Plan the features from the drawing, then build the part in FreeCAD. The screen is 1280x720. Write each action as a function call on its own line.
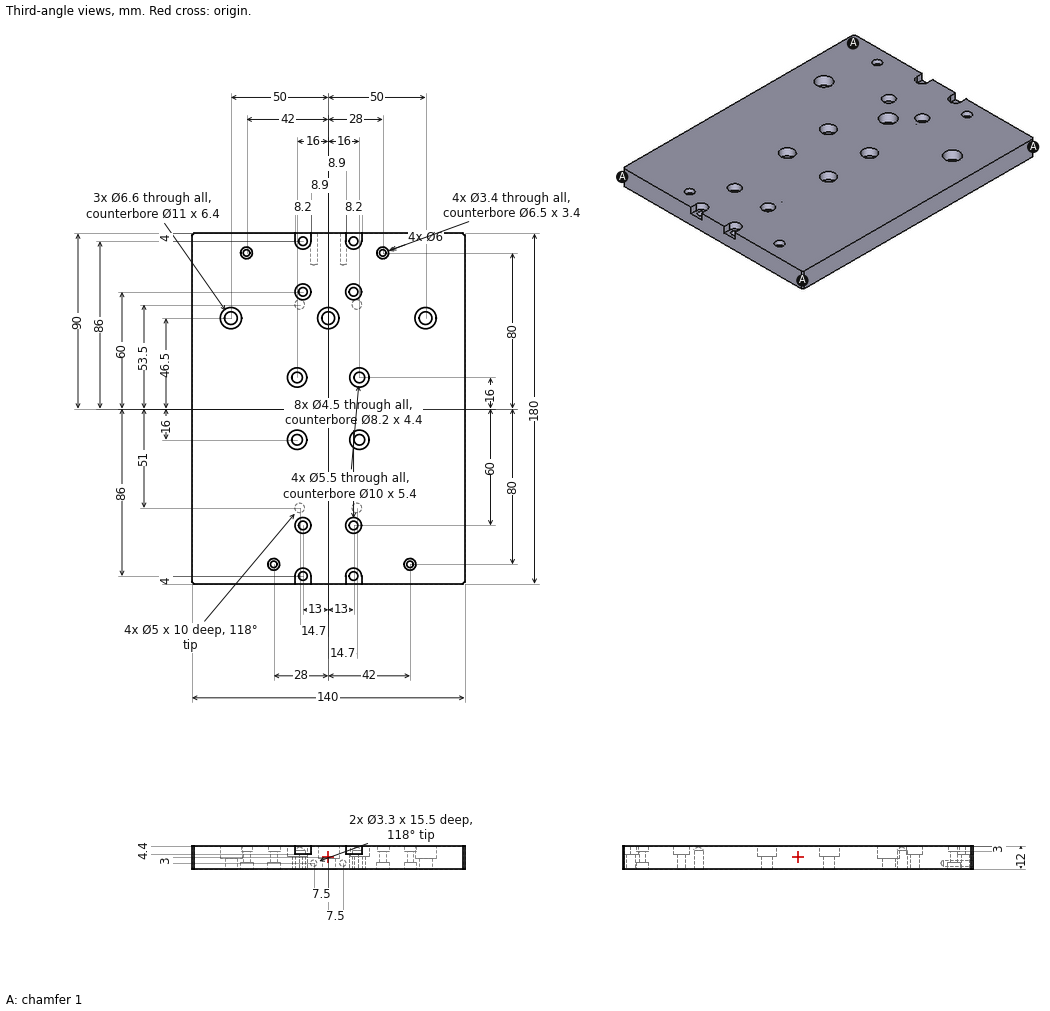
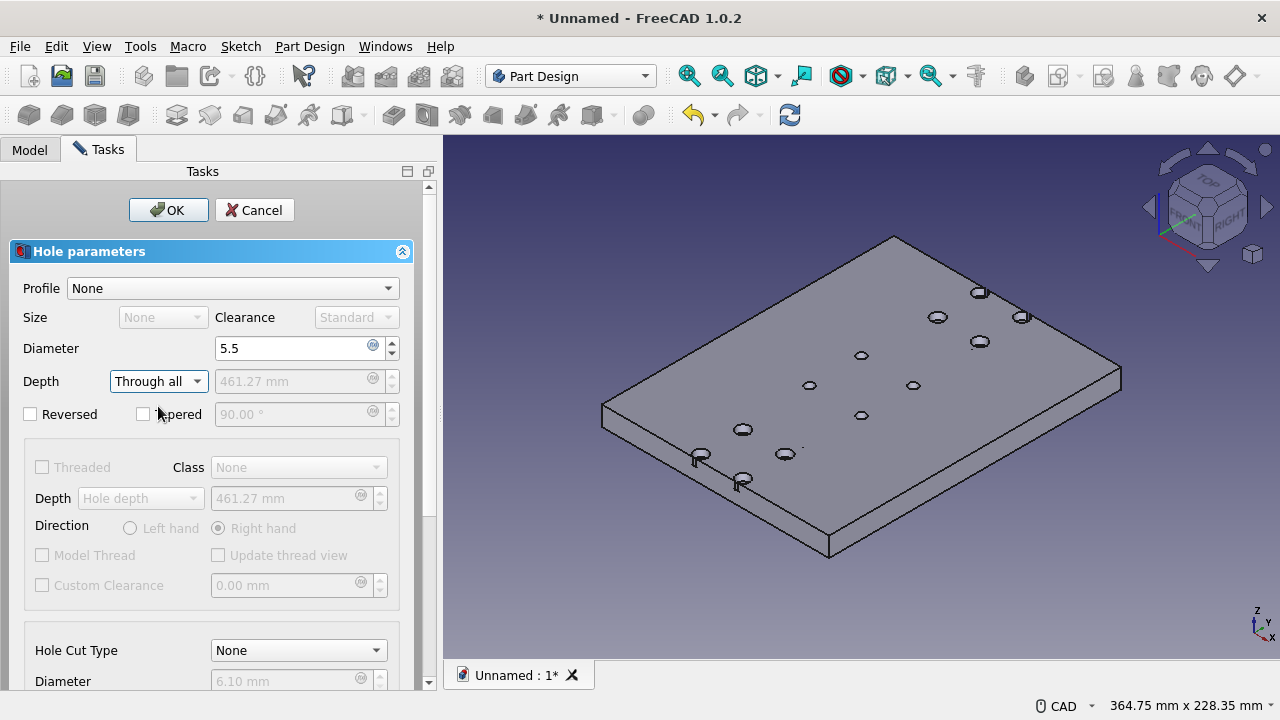
click(300, 650)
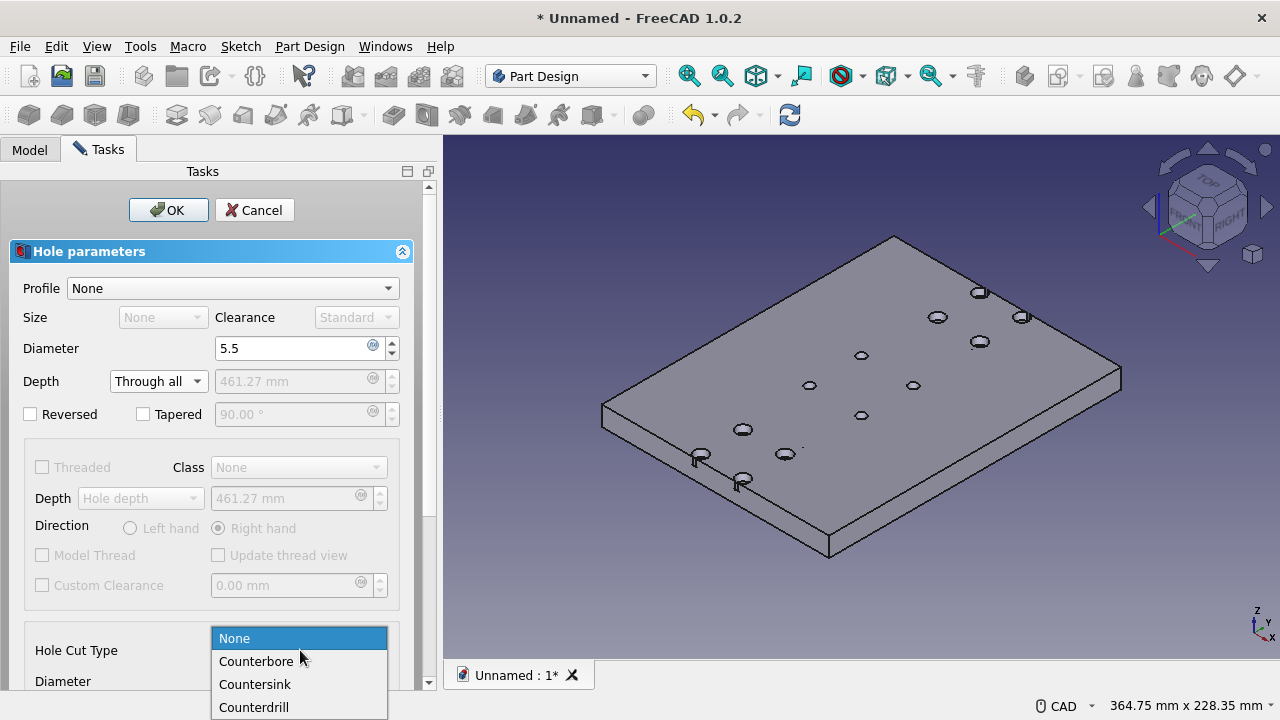
click(298, 662)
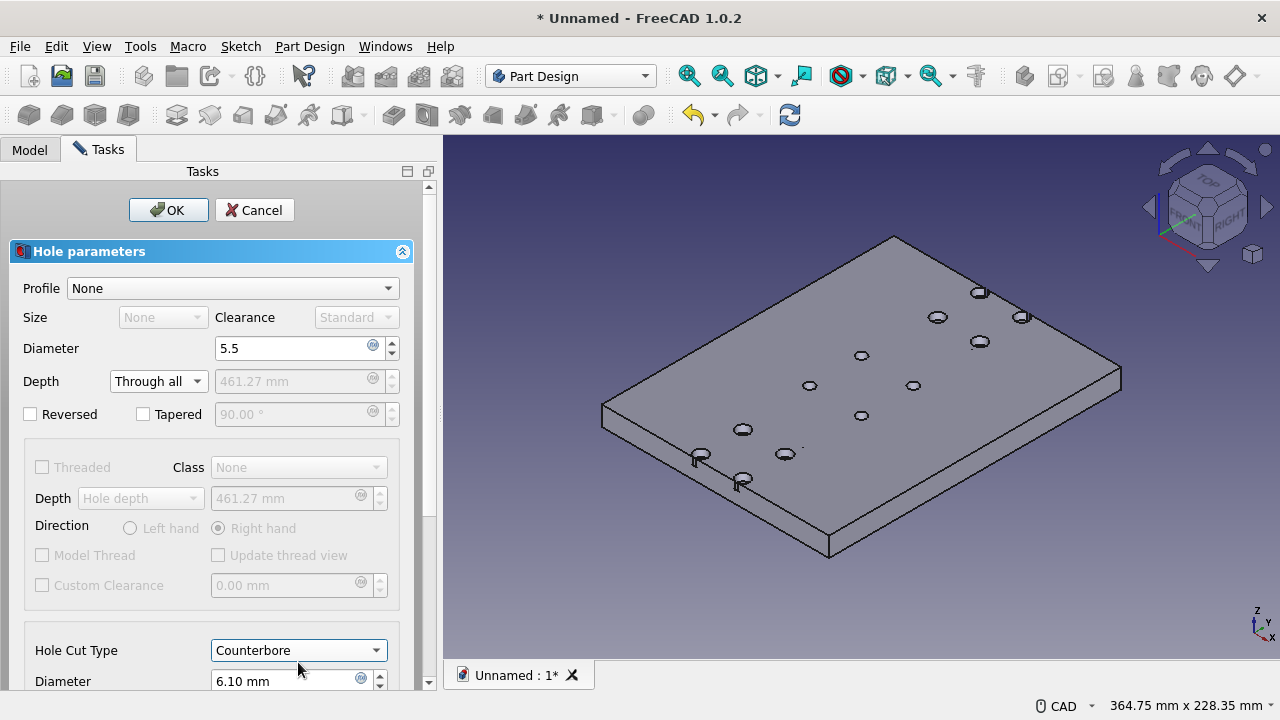
scroll(429, 436, down, 2)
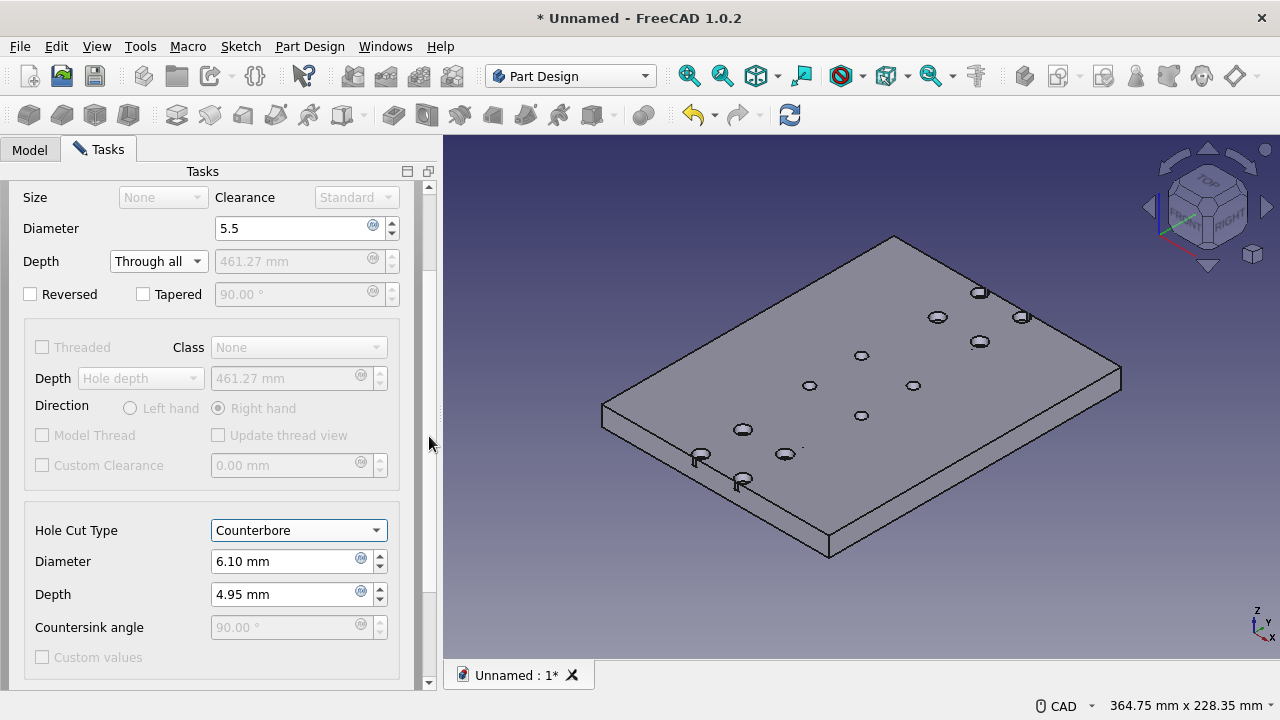
triple_click(292, 562)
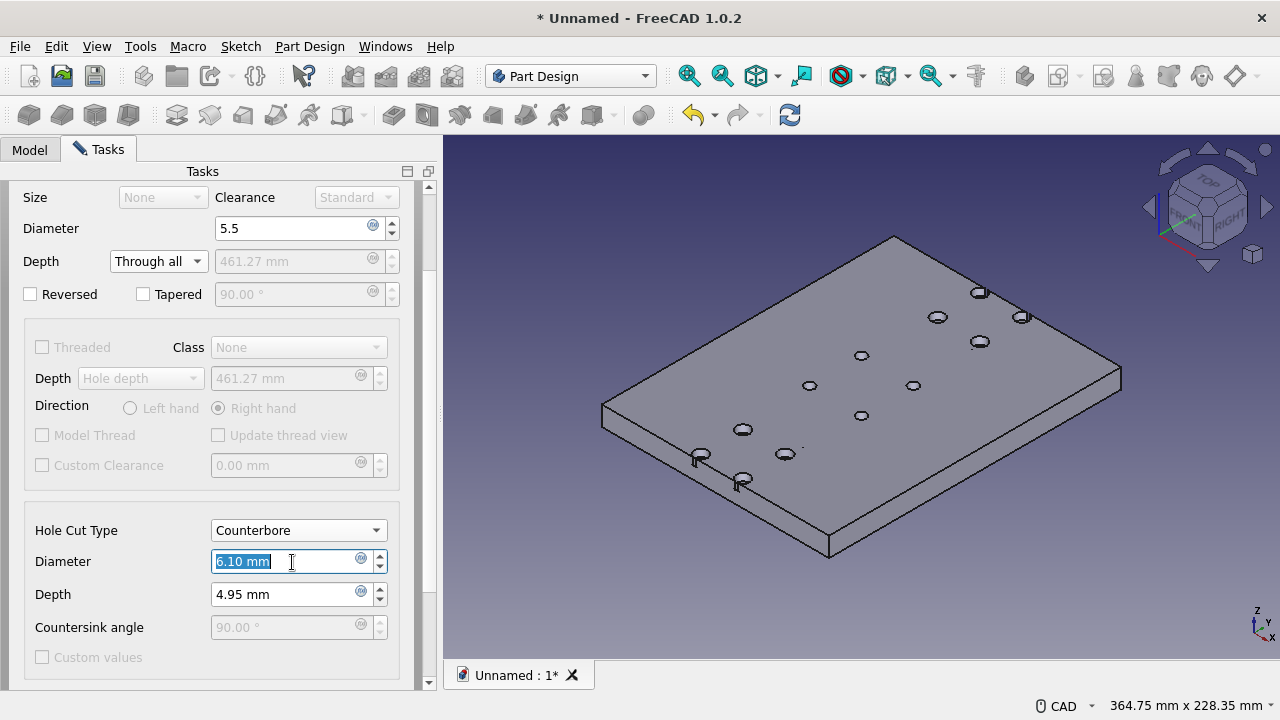
text(10)
key(Tab)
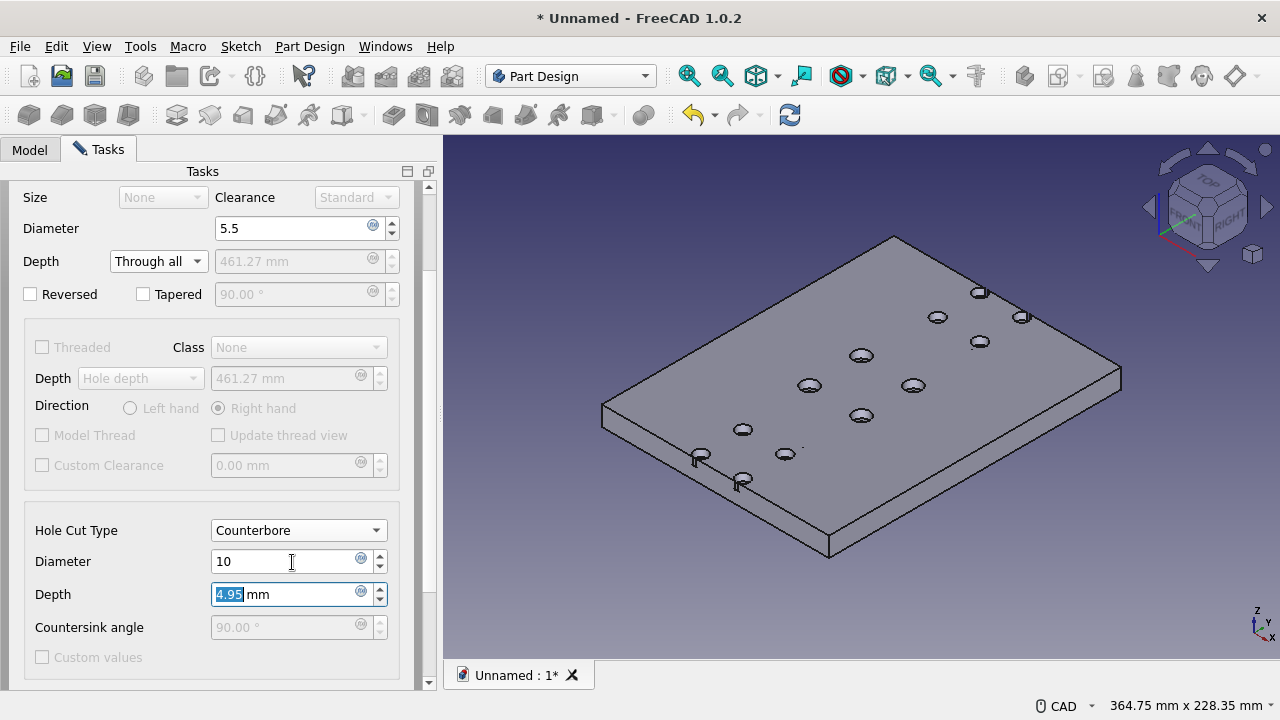
text(5.4)
key(Tab)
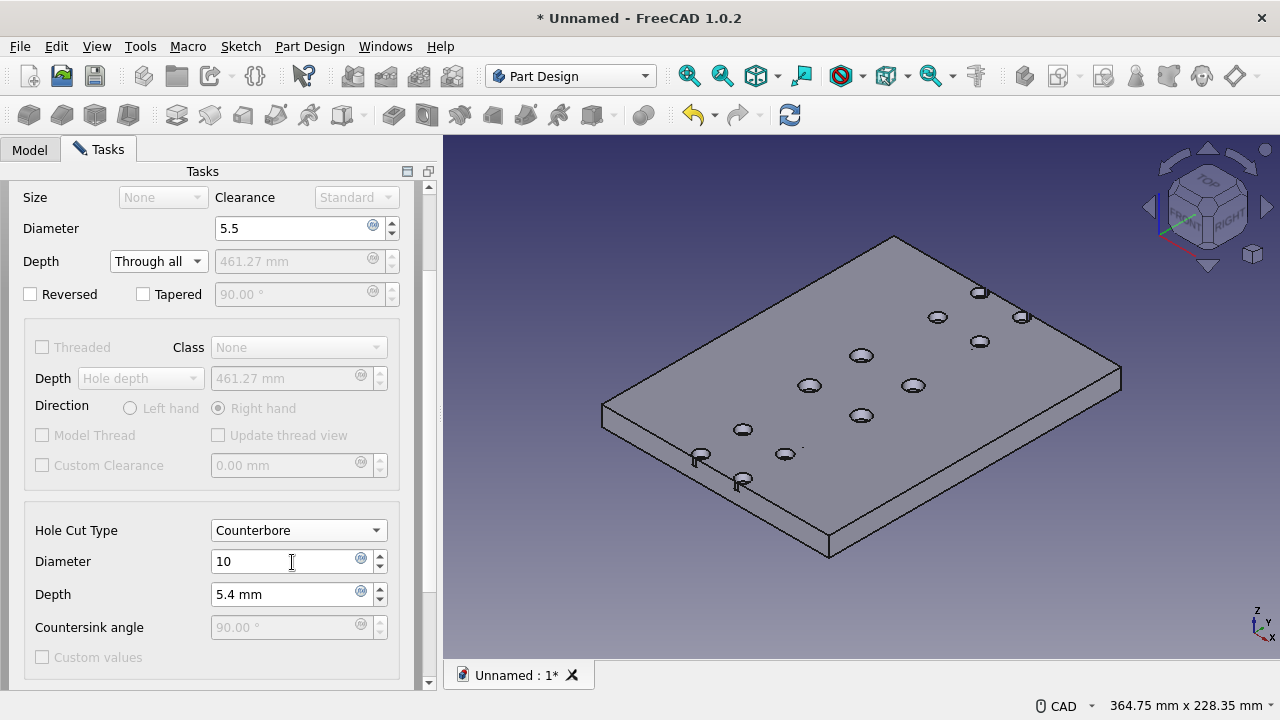
scroll(429, 436, up, 3)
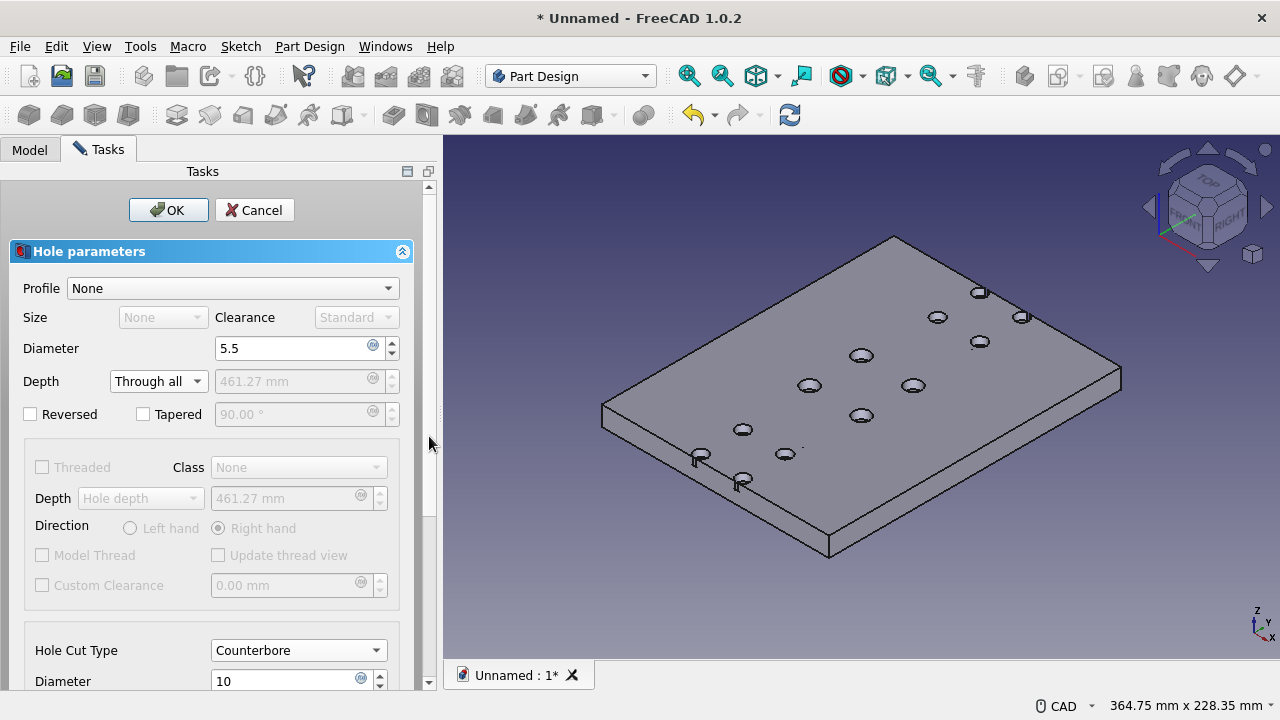
click(169, 210)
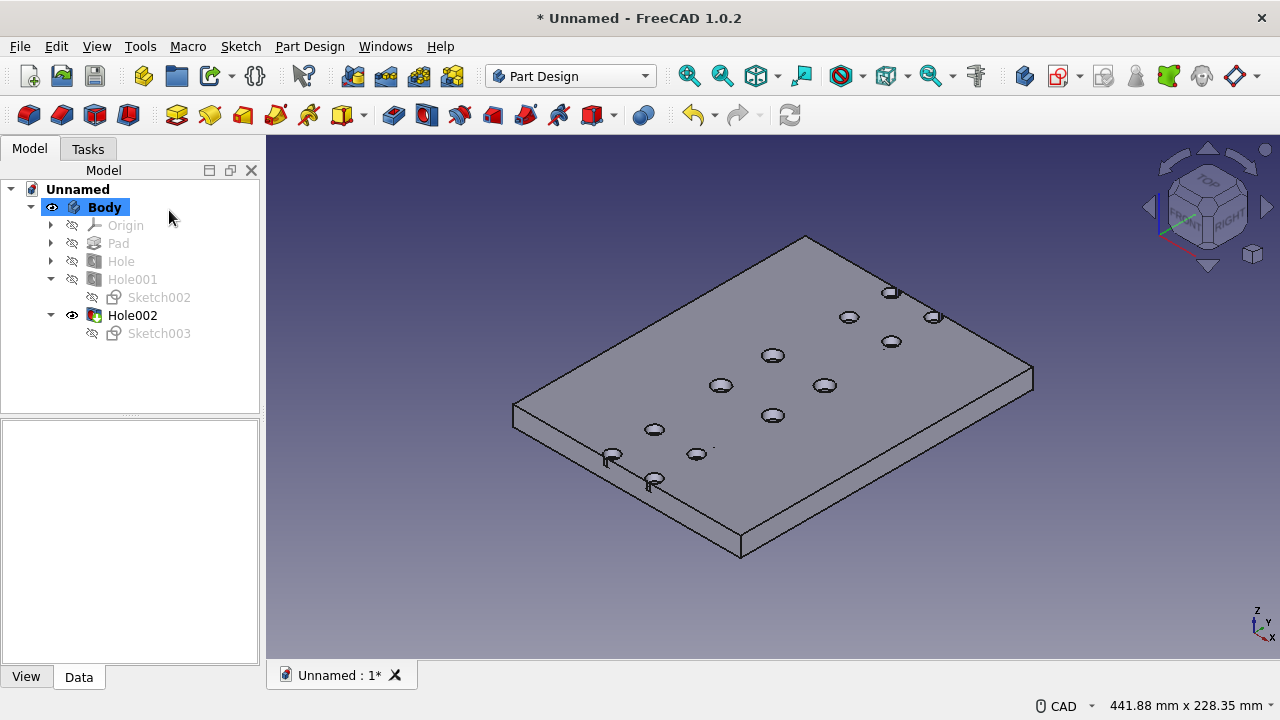
click(921, 374)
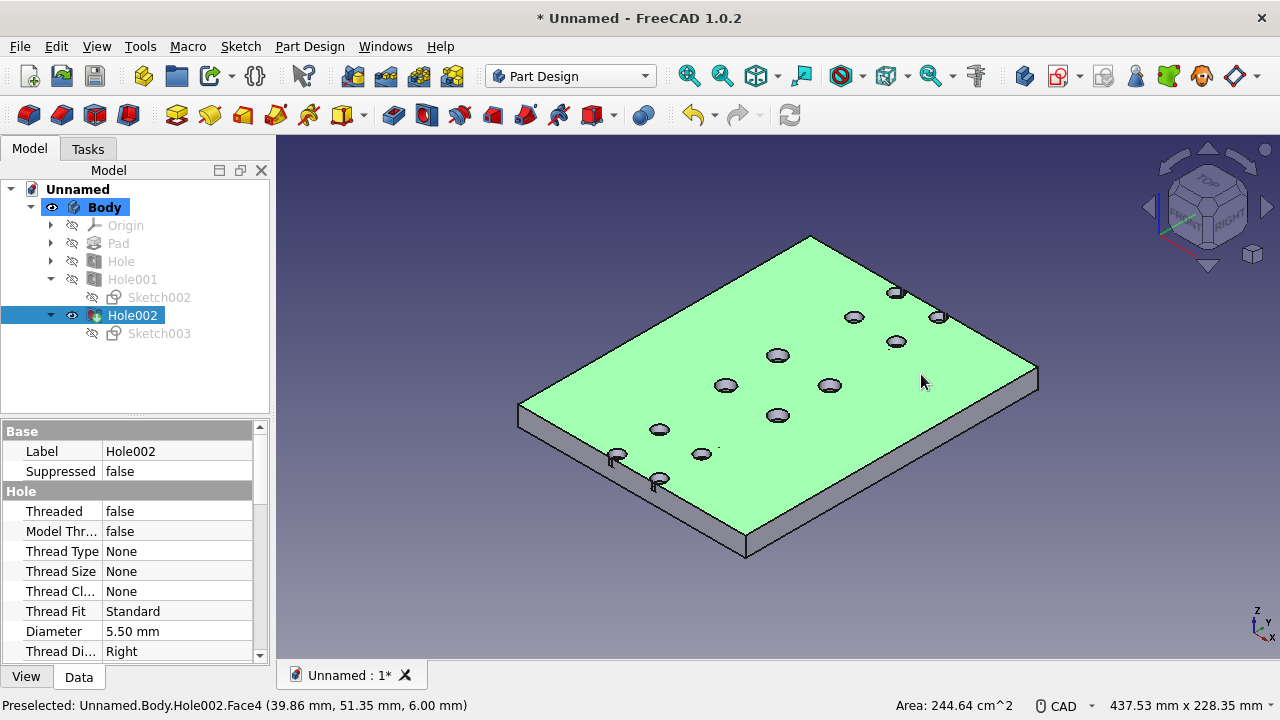
click(1058, 76)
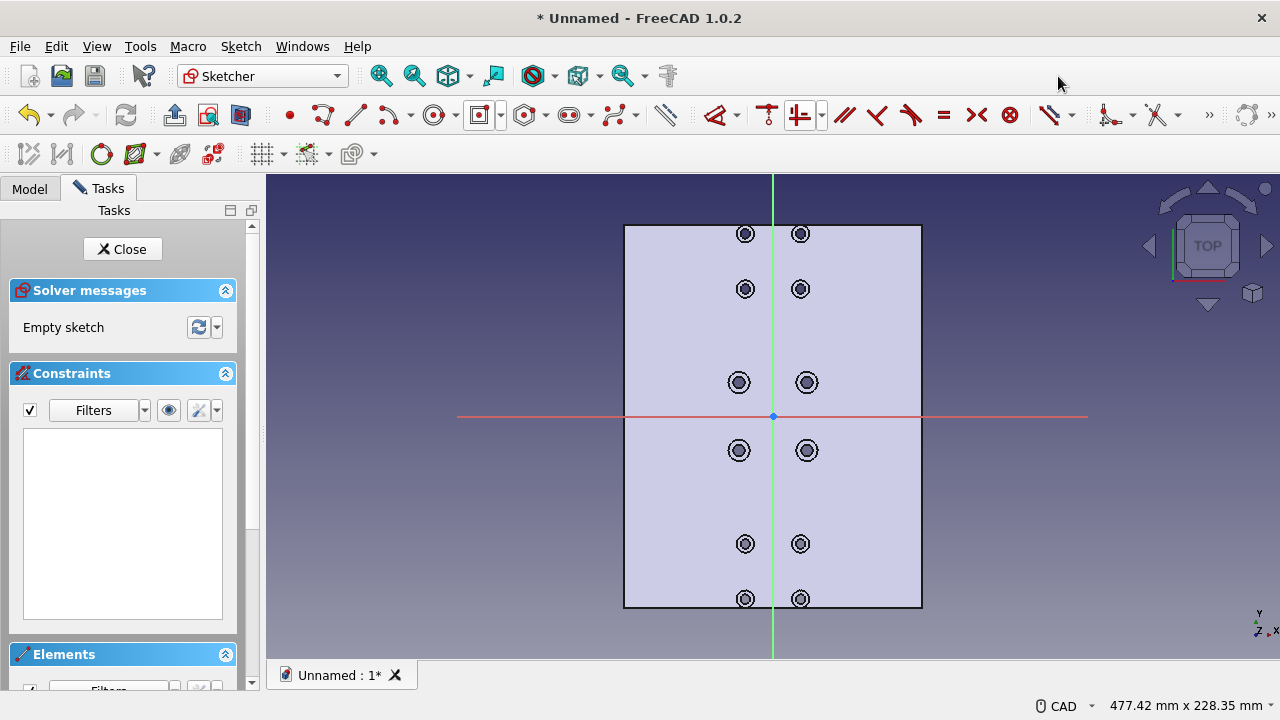
scroll(395, 416, down, 1)